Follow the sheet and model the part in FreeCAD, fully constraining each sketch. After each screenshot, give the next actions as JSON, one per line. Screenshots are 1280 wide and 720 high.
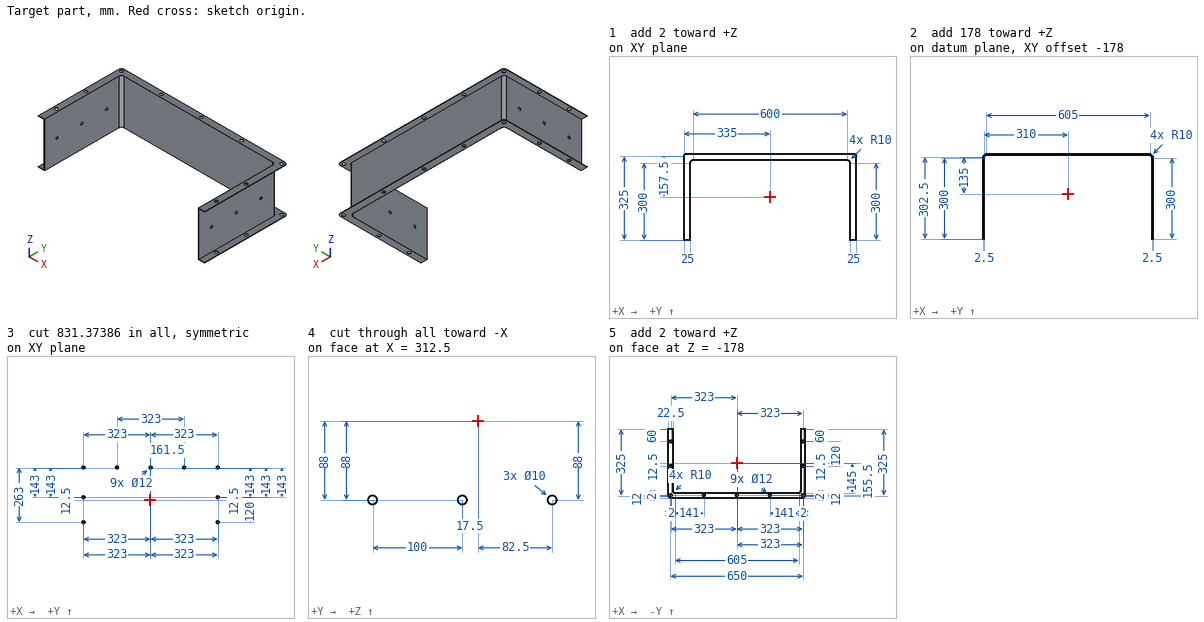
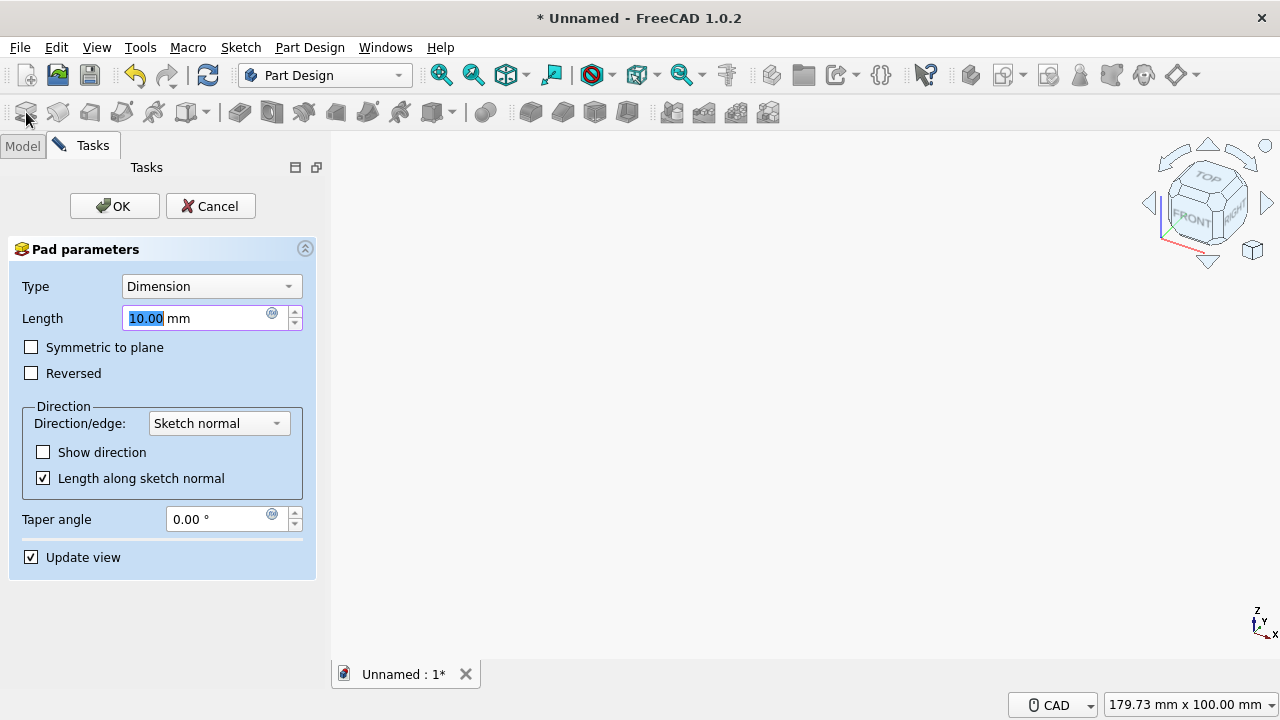
{"action": "type", "text": "2"}
{"action": "key", "text": "Tab"}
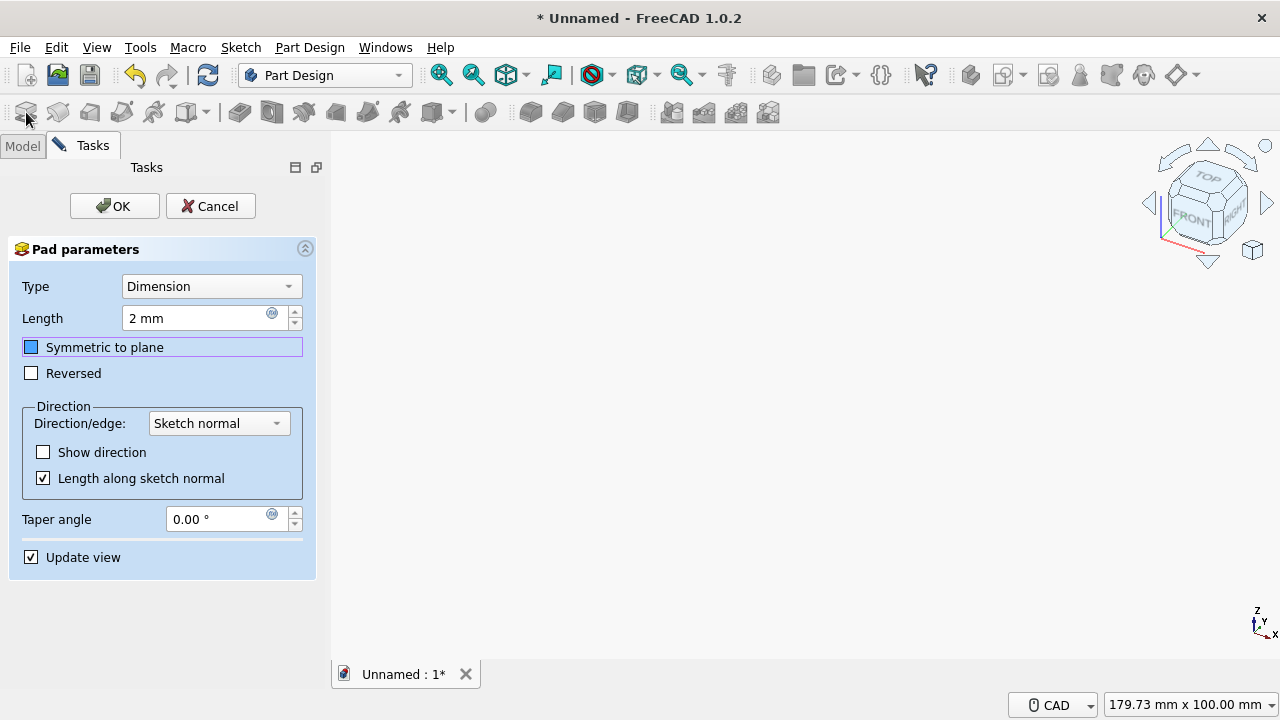
{"action": "left_click", "coordinate": [115, 206]}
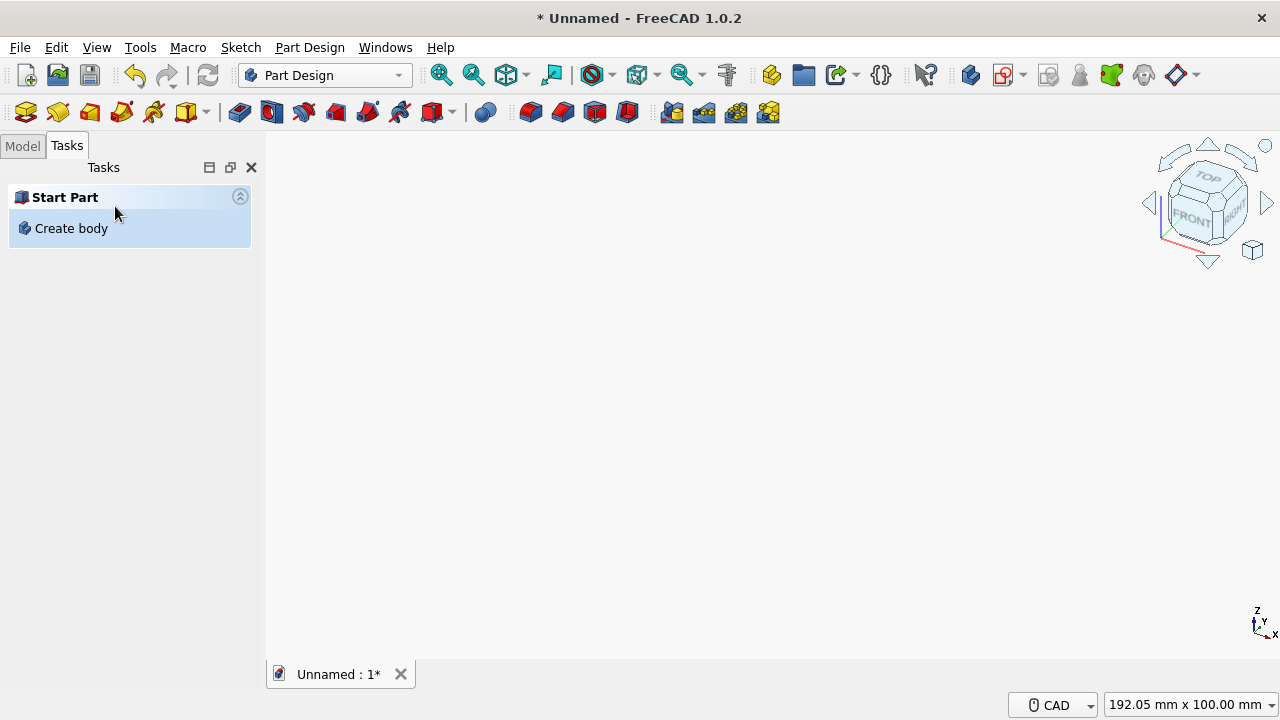
{"action": "key", "text": "v f"}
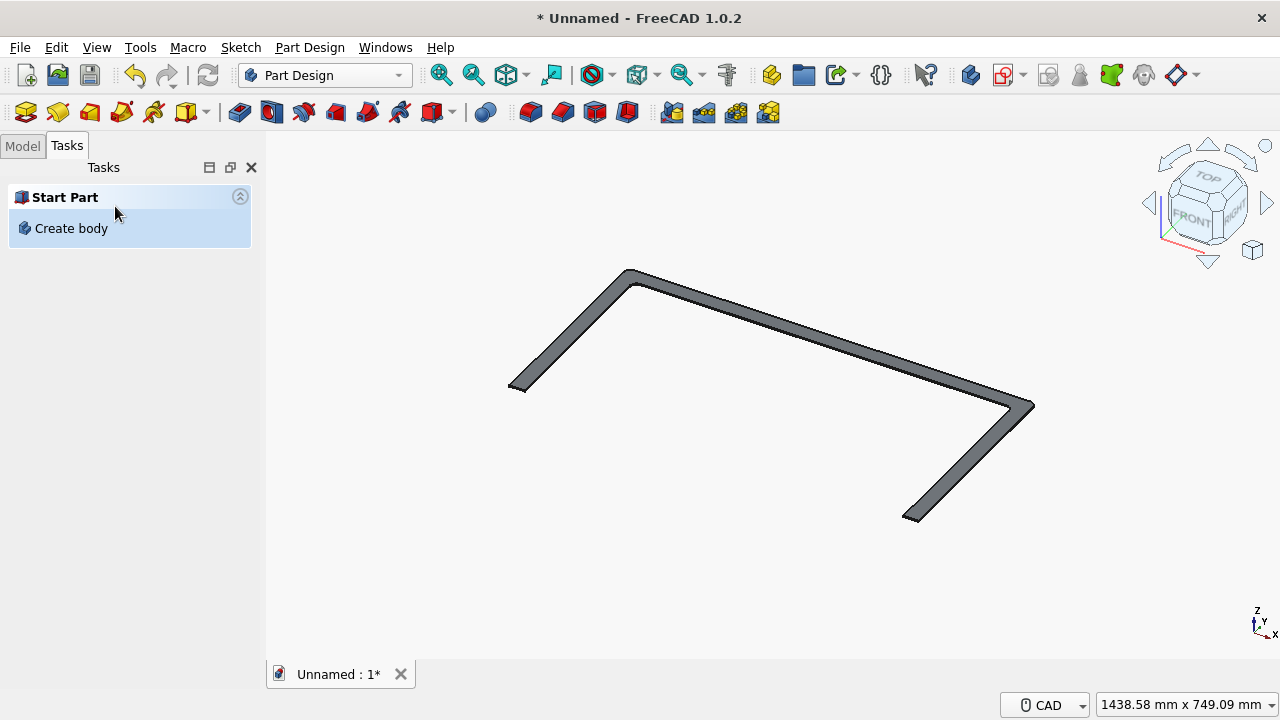
{"action": "left_click", "coordinate": [23, 145]}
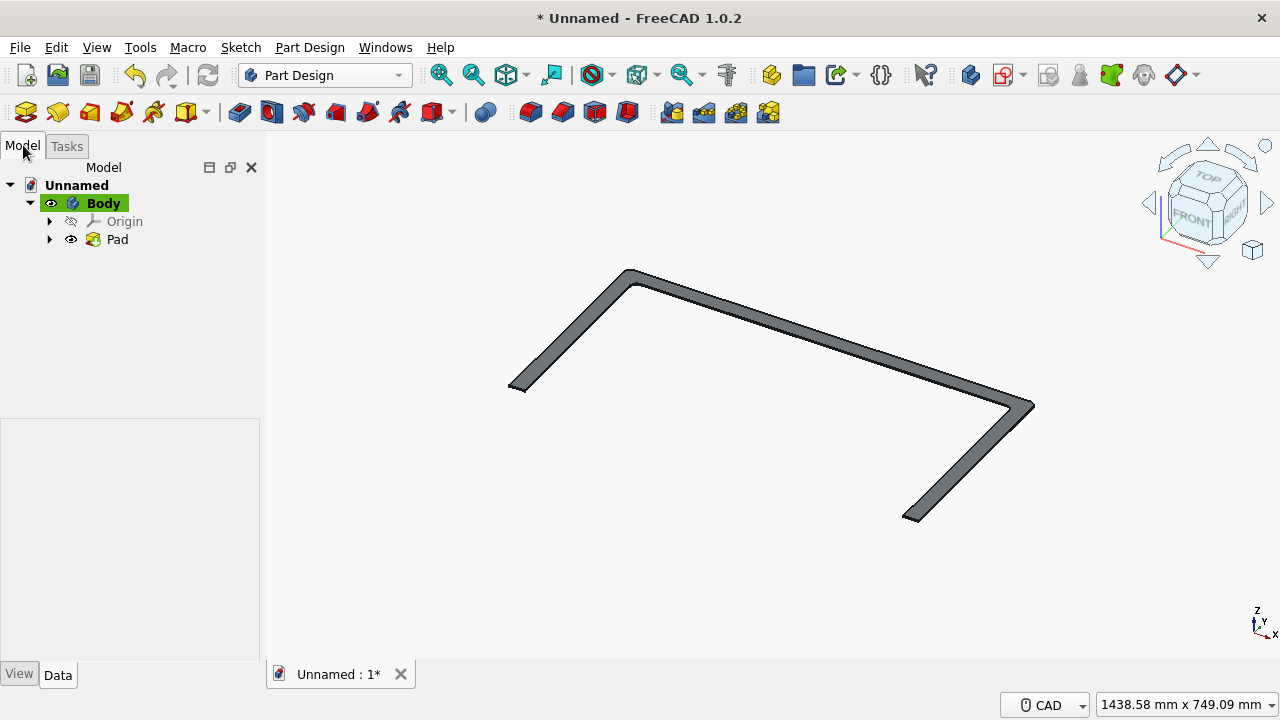
{"action": "left_click", "coordinate": [50, 221]}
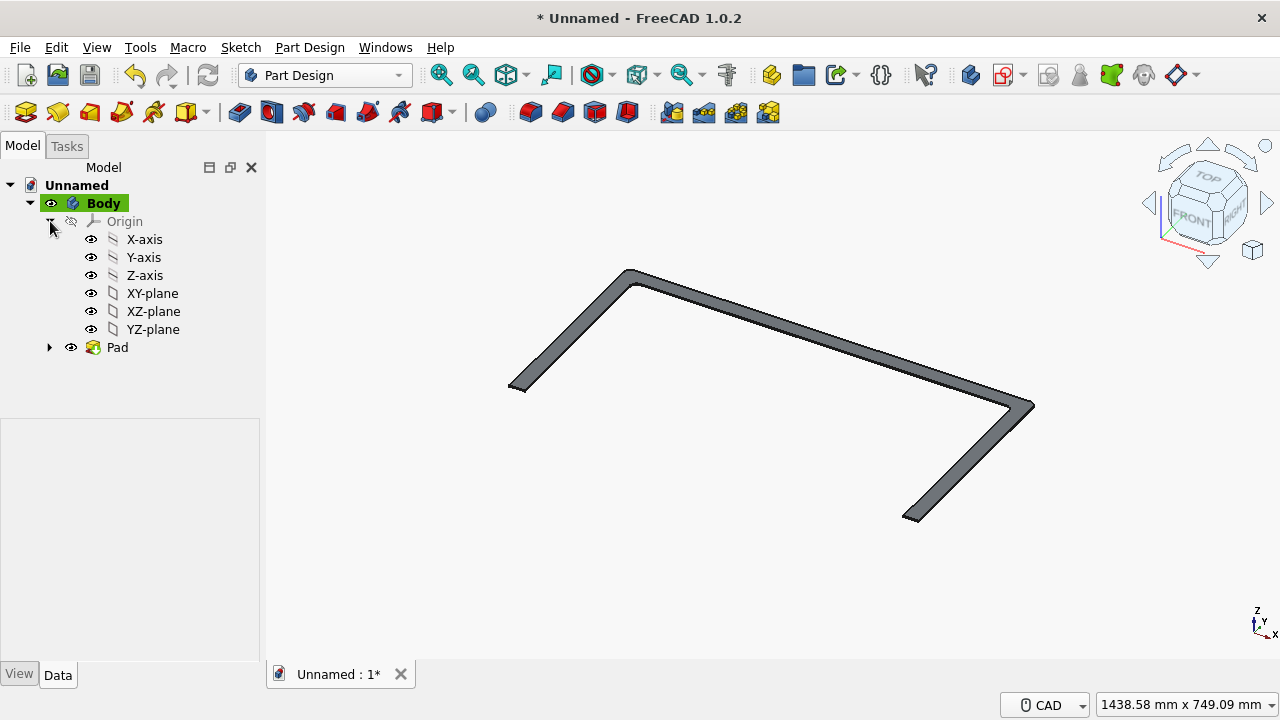
{"action": "left_click", "coordinate": [136, 293]}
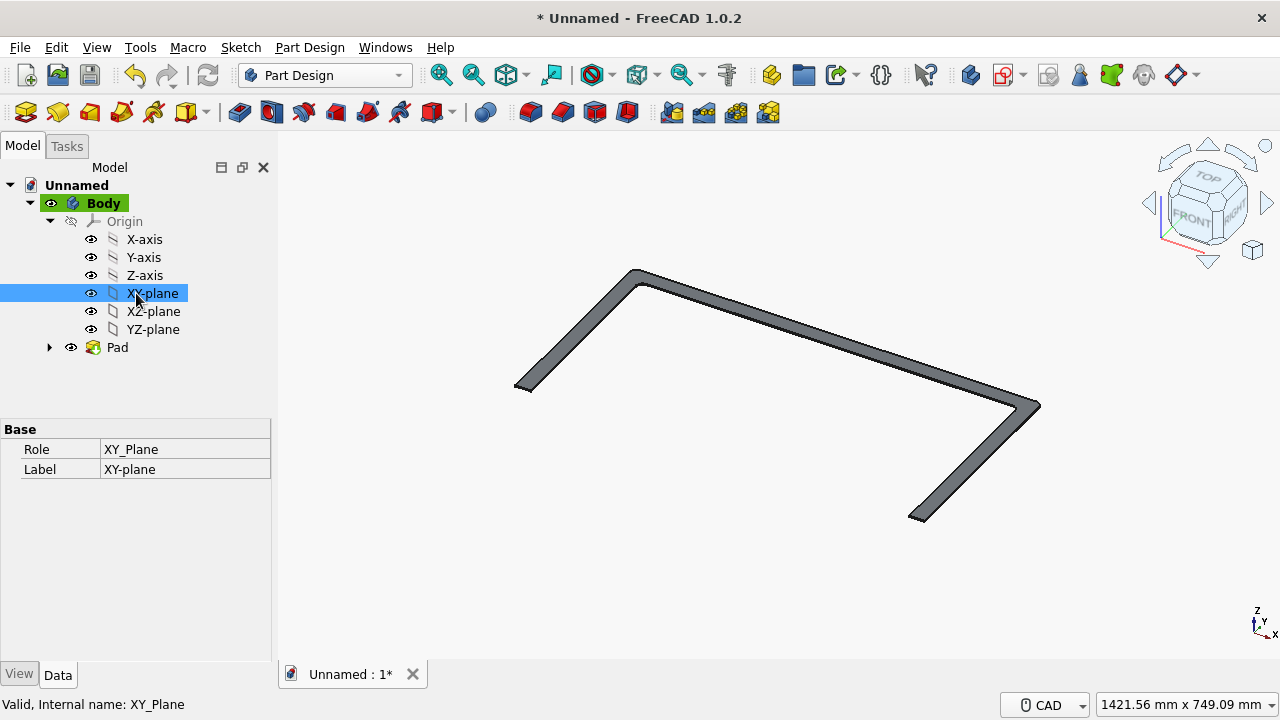
{"action": "left_click", "coordinate": [1176, 76]}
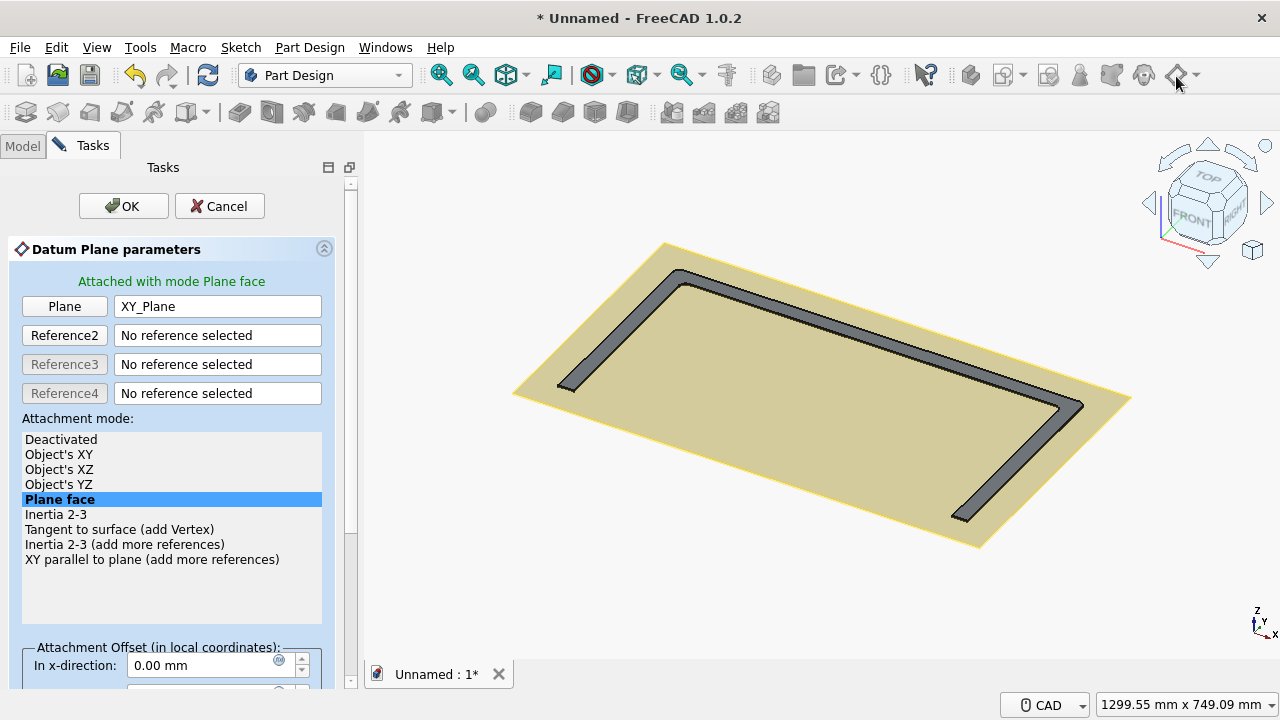
{"action": "scroll", "coordinate": [351, 432], "scroll_direction": "down", "scroll_amount": 2}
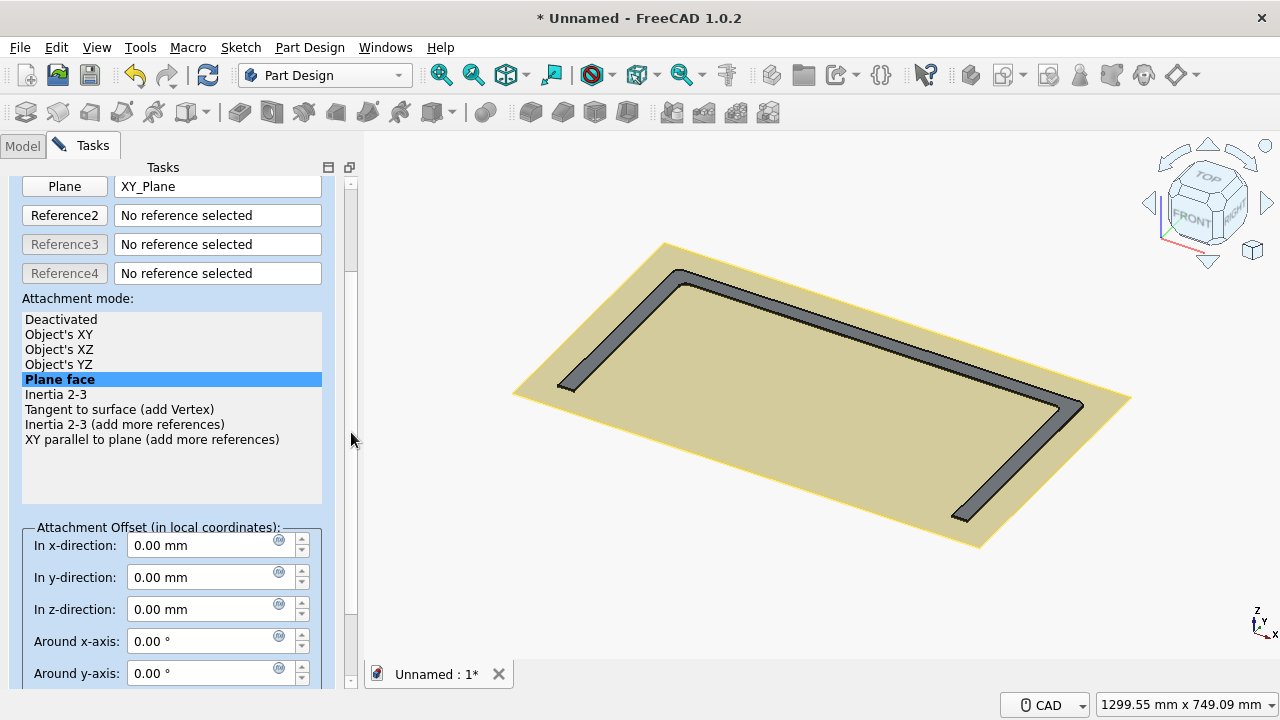
{"action": "triple_click", "coordinate": [210, 609]}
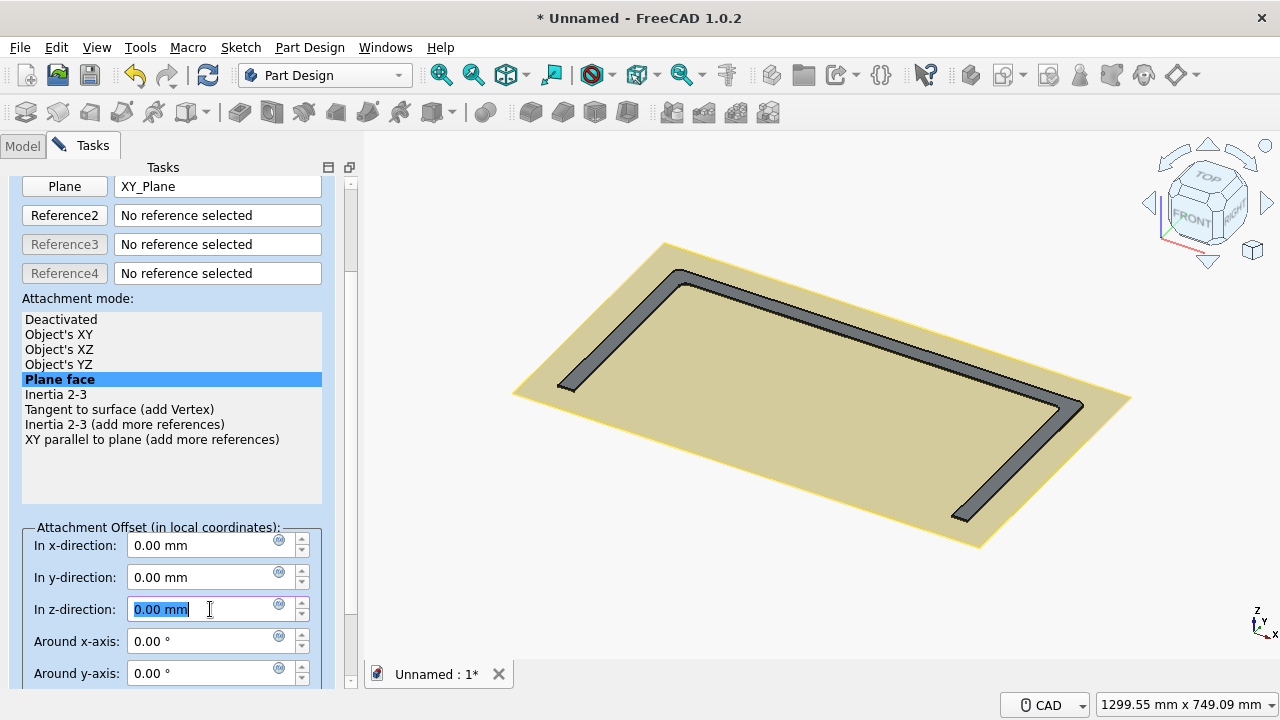
{"action": "type", "text": "-178"}
{"action": "key", "text": "Tab"}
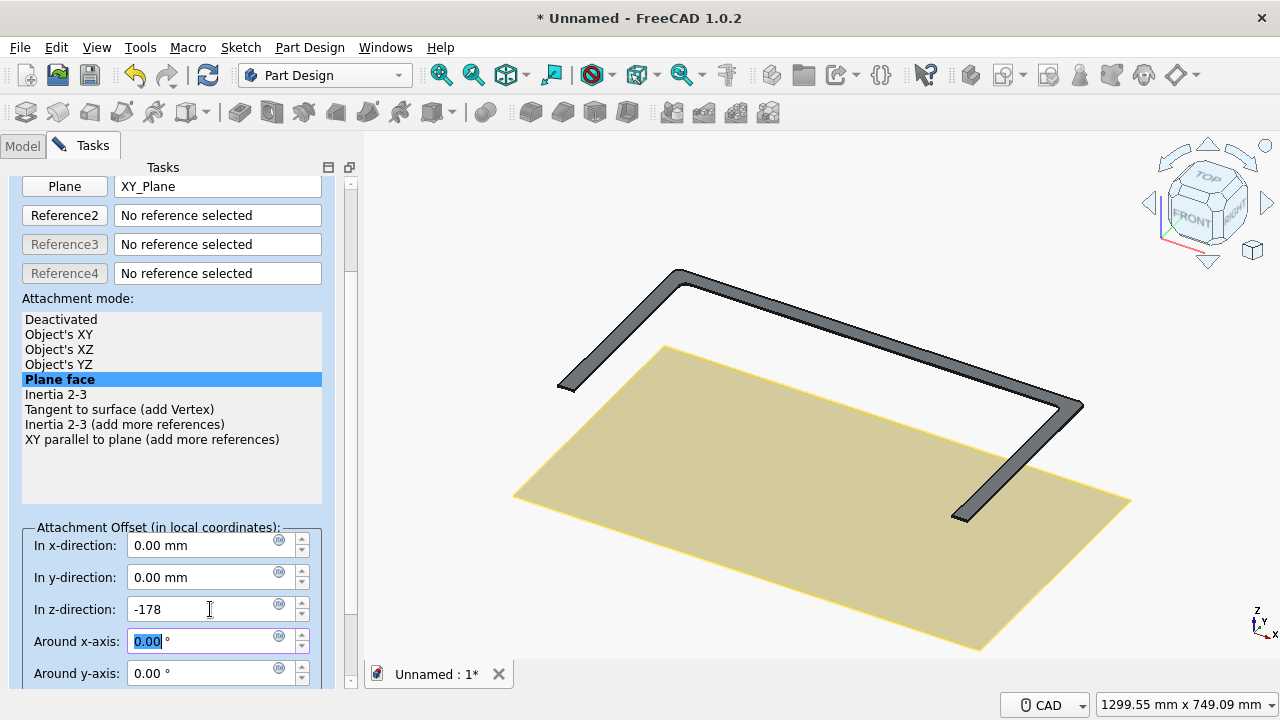
{"action": "scroll", "coordinate": [351, 432], "scroll_direction": "up", "scroll_amount": 3}